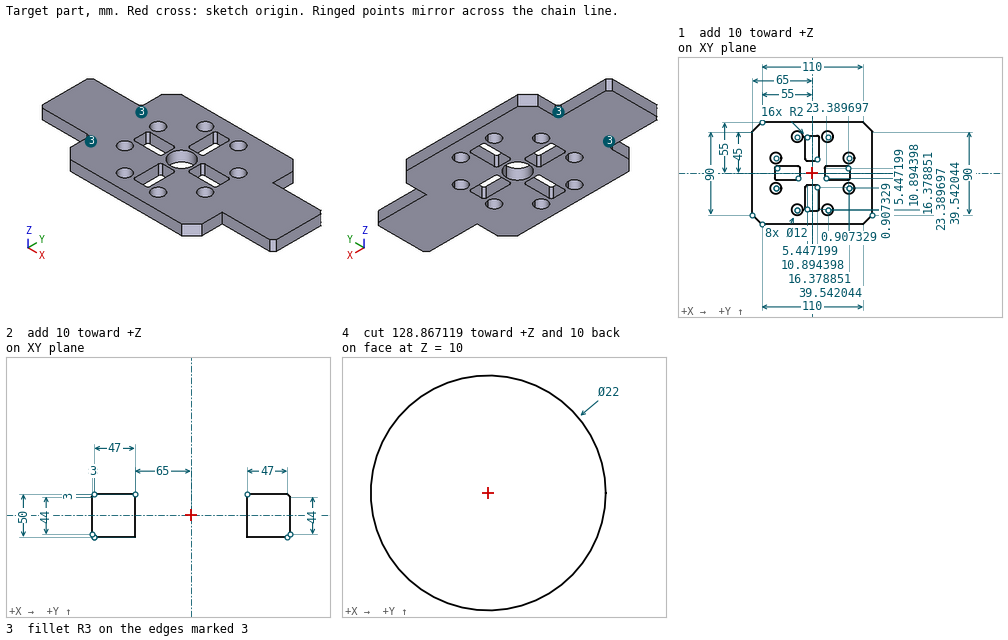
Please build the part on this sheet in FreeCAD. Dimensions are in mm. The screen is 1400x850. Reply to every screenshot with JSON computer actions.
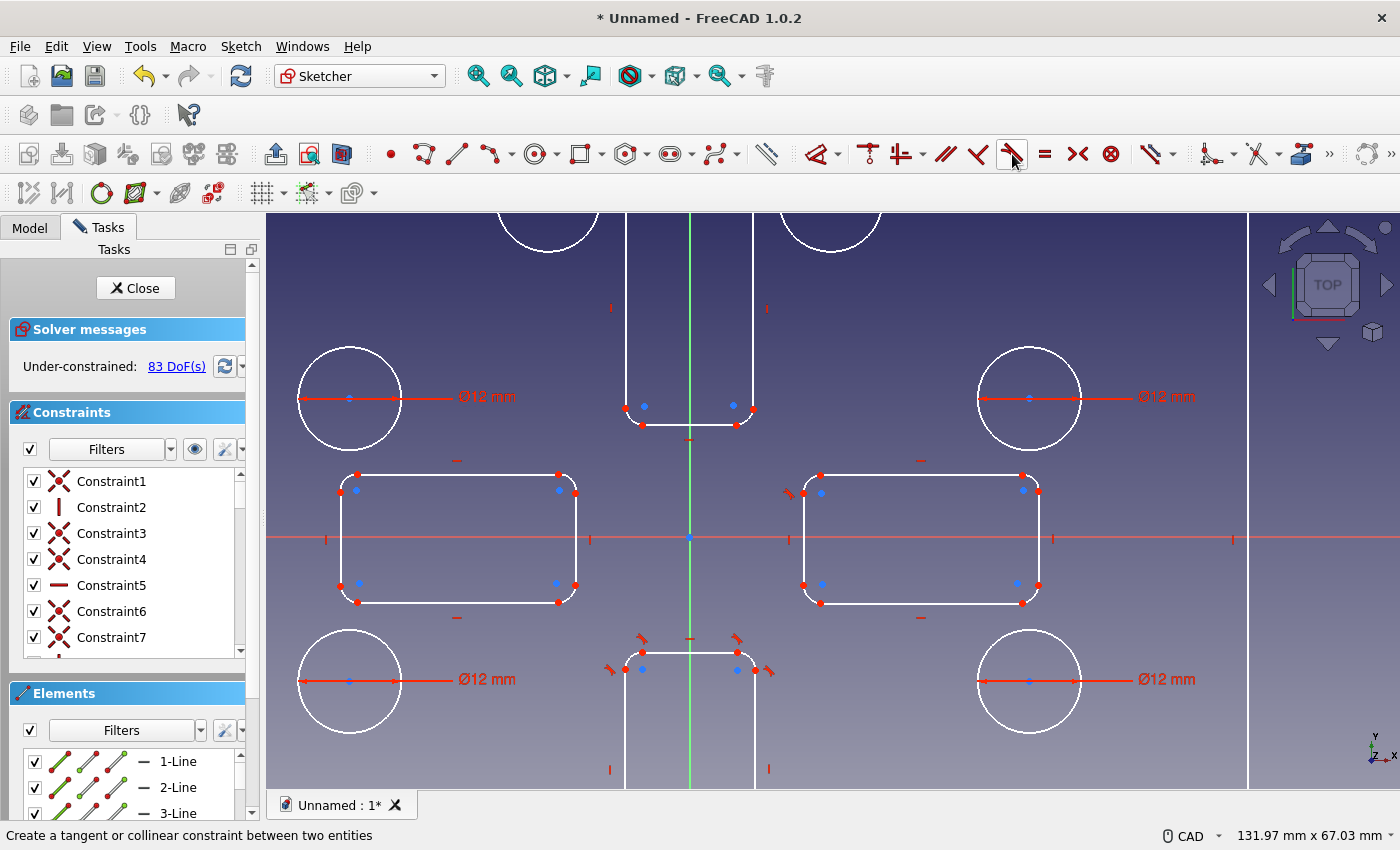
{"action": "left_click", "coordinate": [804, 558]}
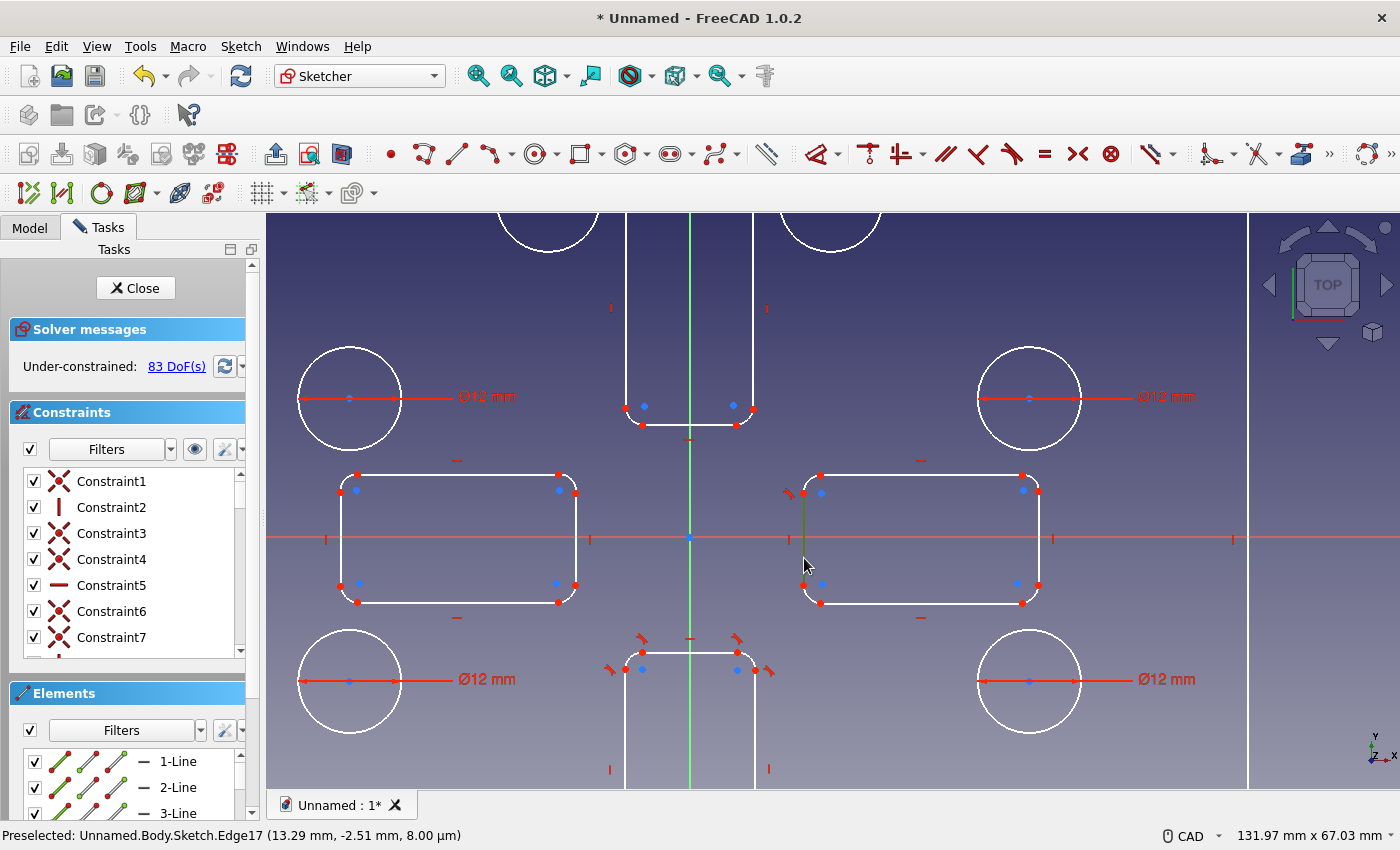
{"action": "left_click", "coordinate": [809, 598]}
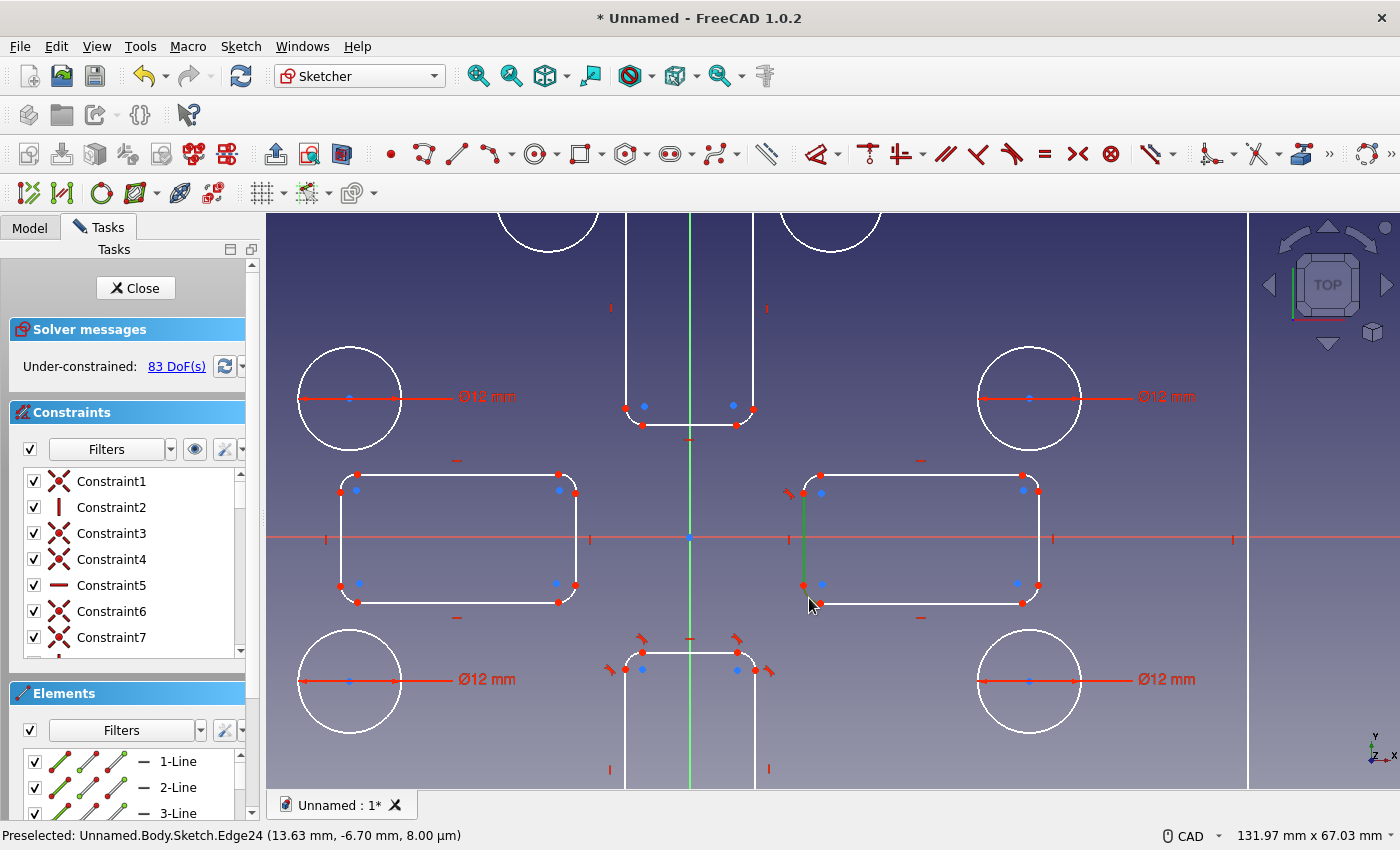
{"action": "left_click", "coordinate": [1012, 154]}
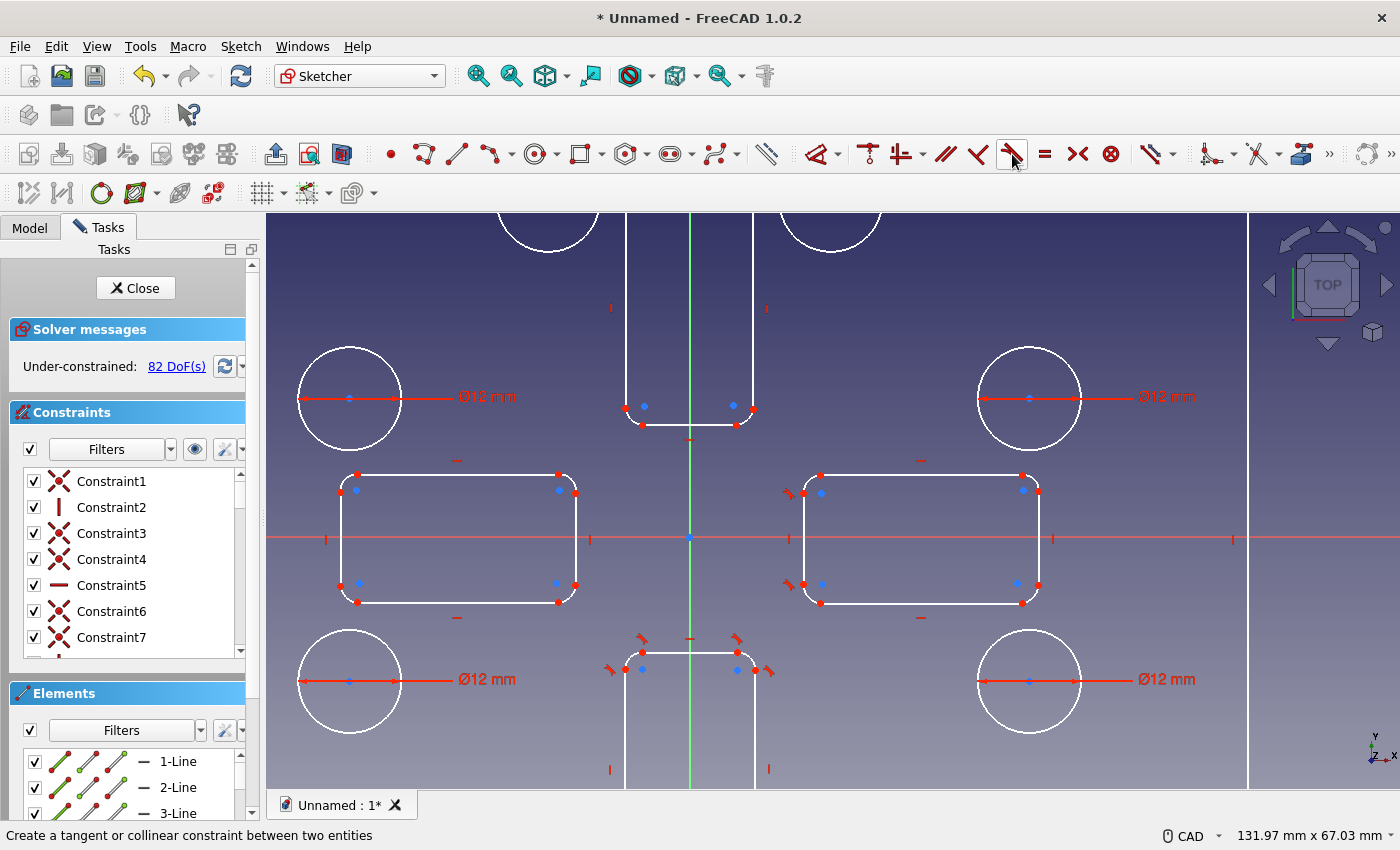
{"action": "left_click", "coordinate": [881, 475]}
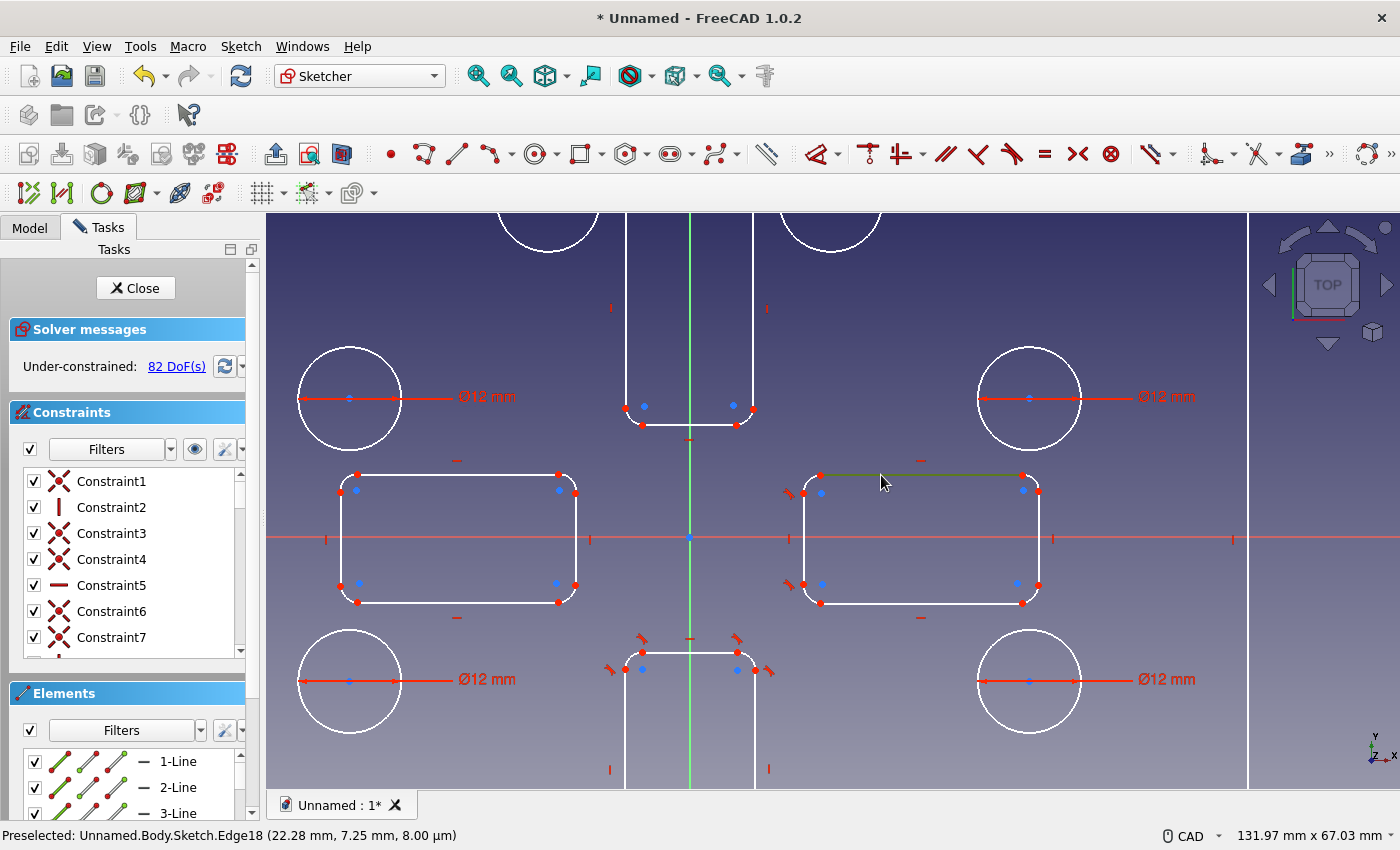
{"action": "left_click", "coordinate": [809, 481]}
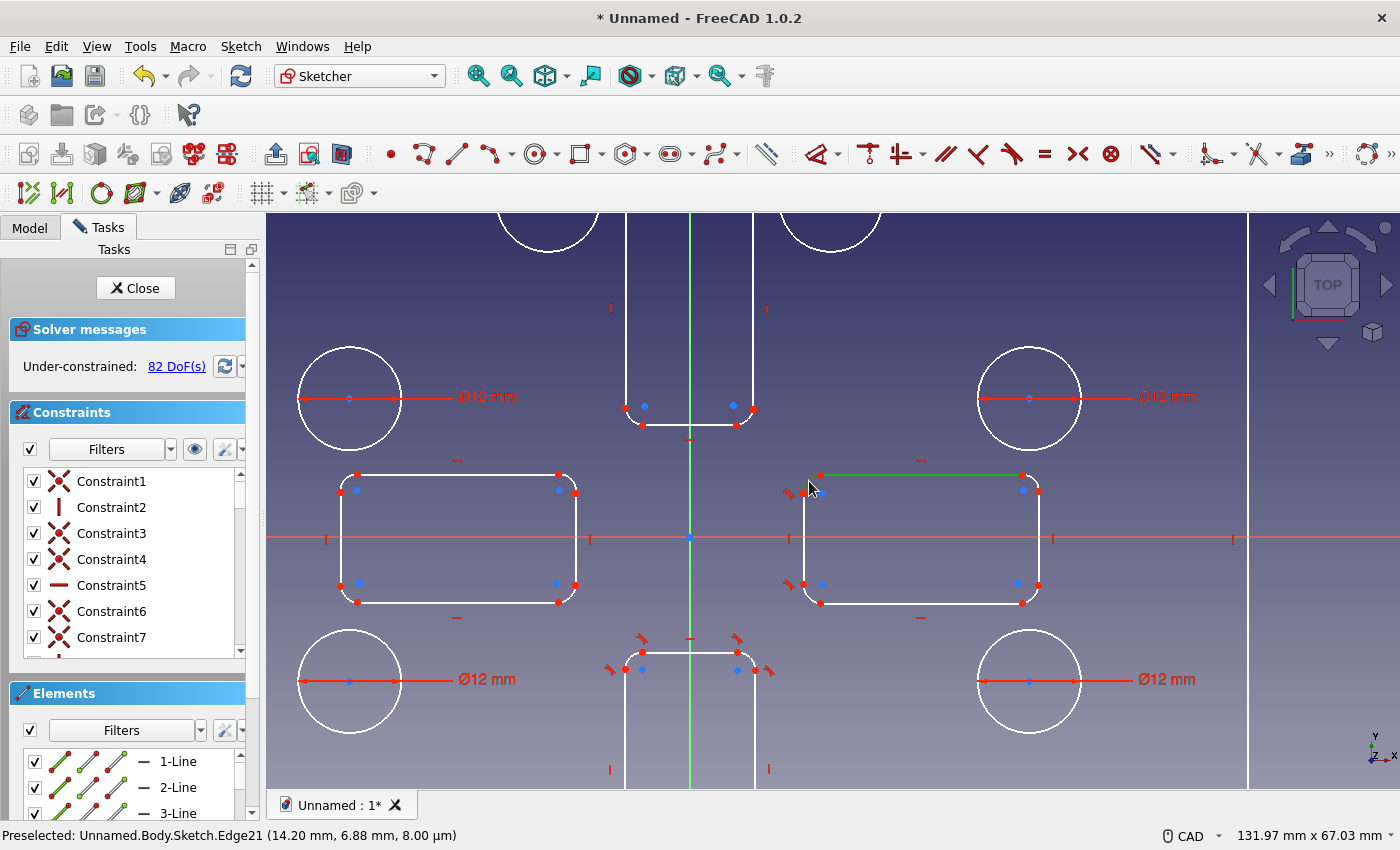
{"action": "left_click", "coordinate": [1012, 154]}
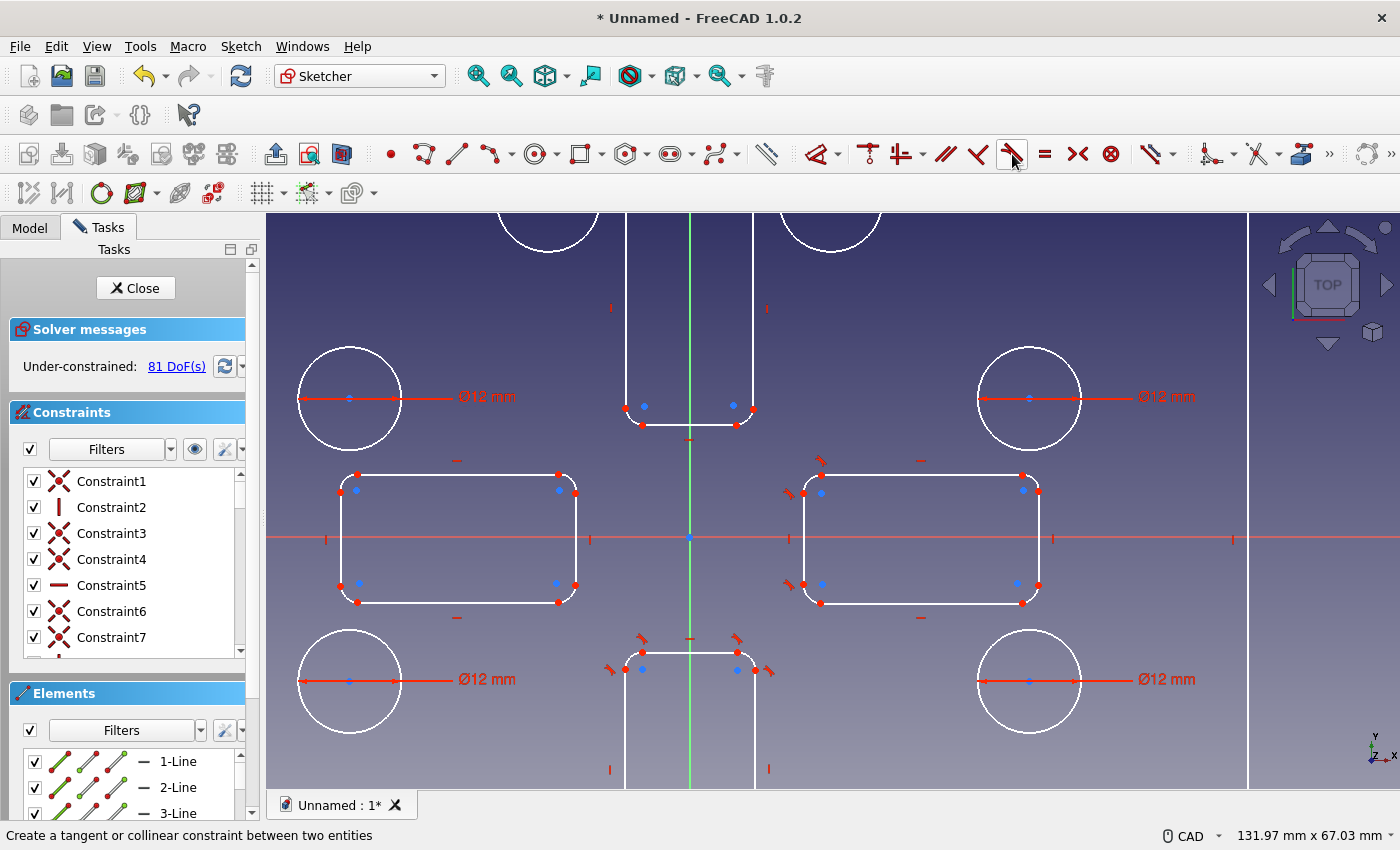
{"action": "left_click", "coordinate": [882, 475]}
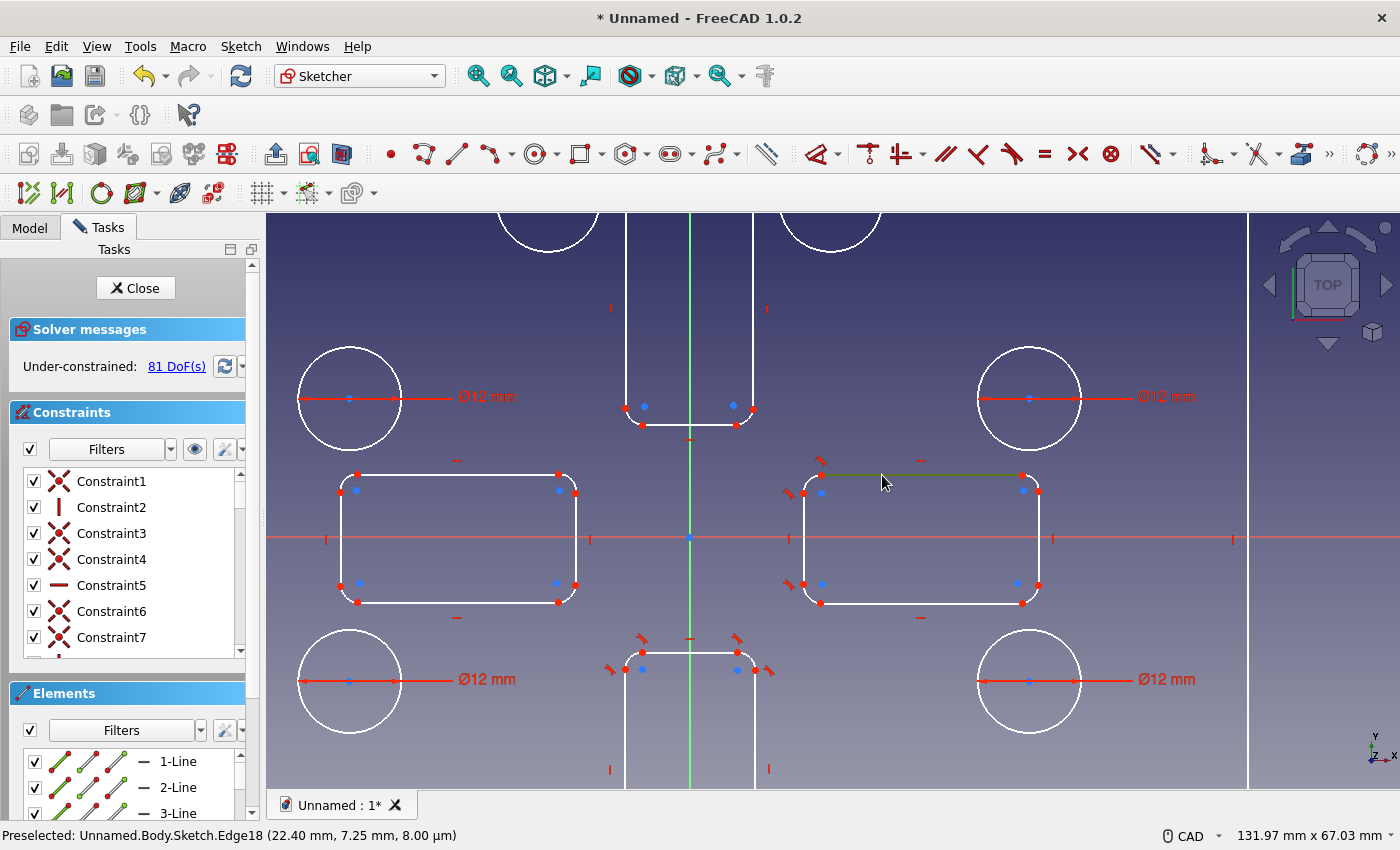
{"action": "left_click", "coordinate": [1034, 479]}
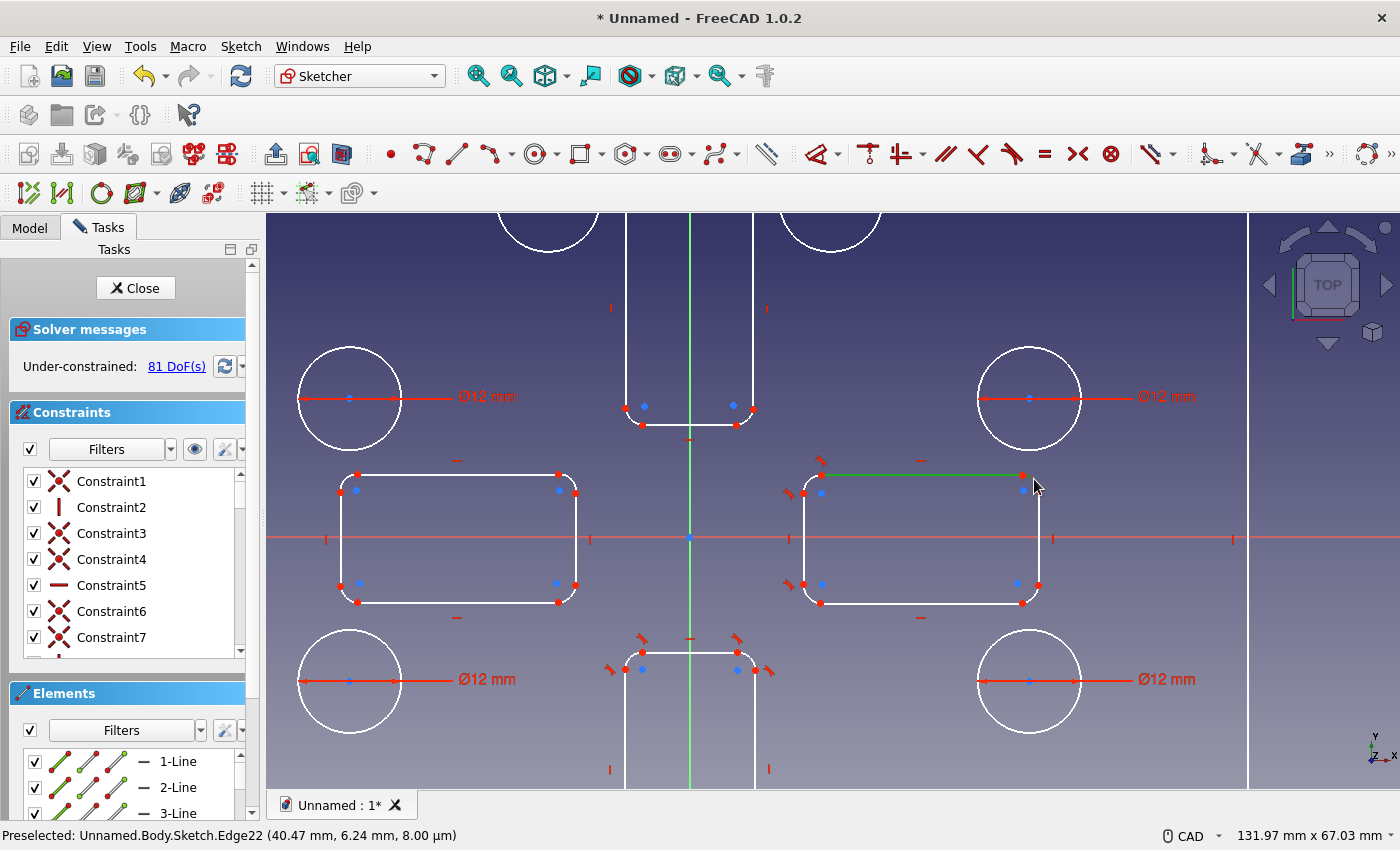
{"action": "left_click", "coordinate": [1012, 154]}